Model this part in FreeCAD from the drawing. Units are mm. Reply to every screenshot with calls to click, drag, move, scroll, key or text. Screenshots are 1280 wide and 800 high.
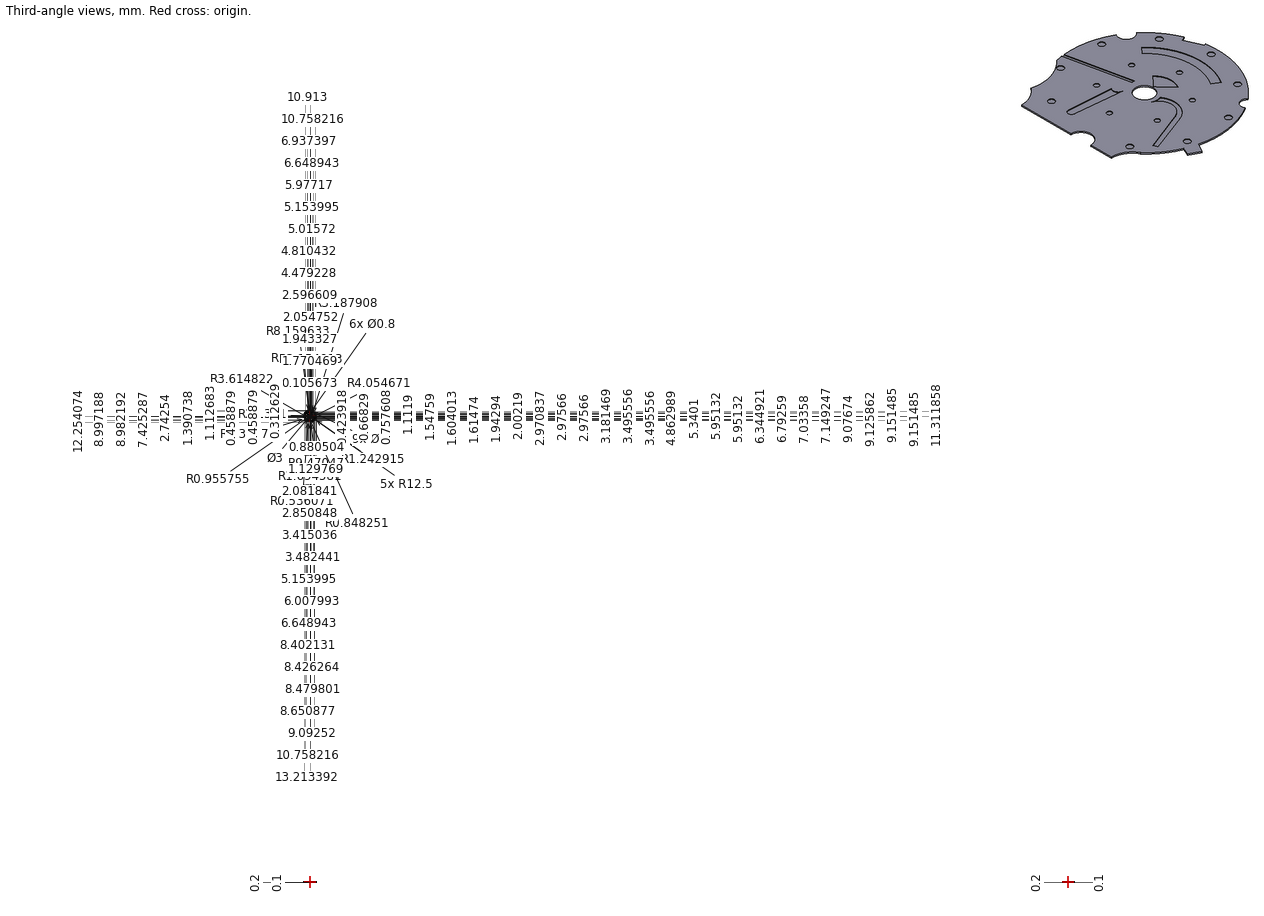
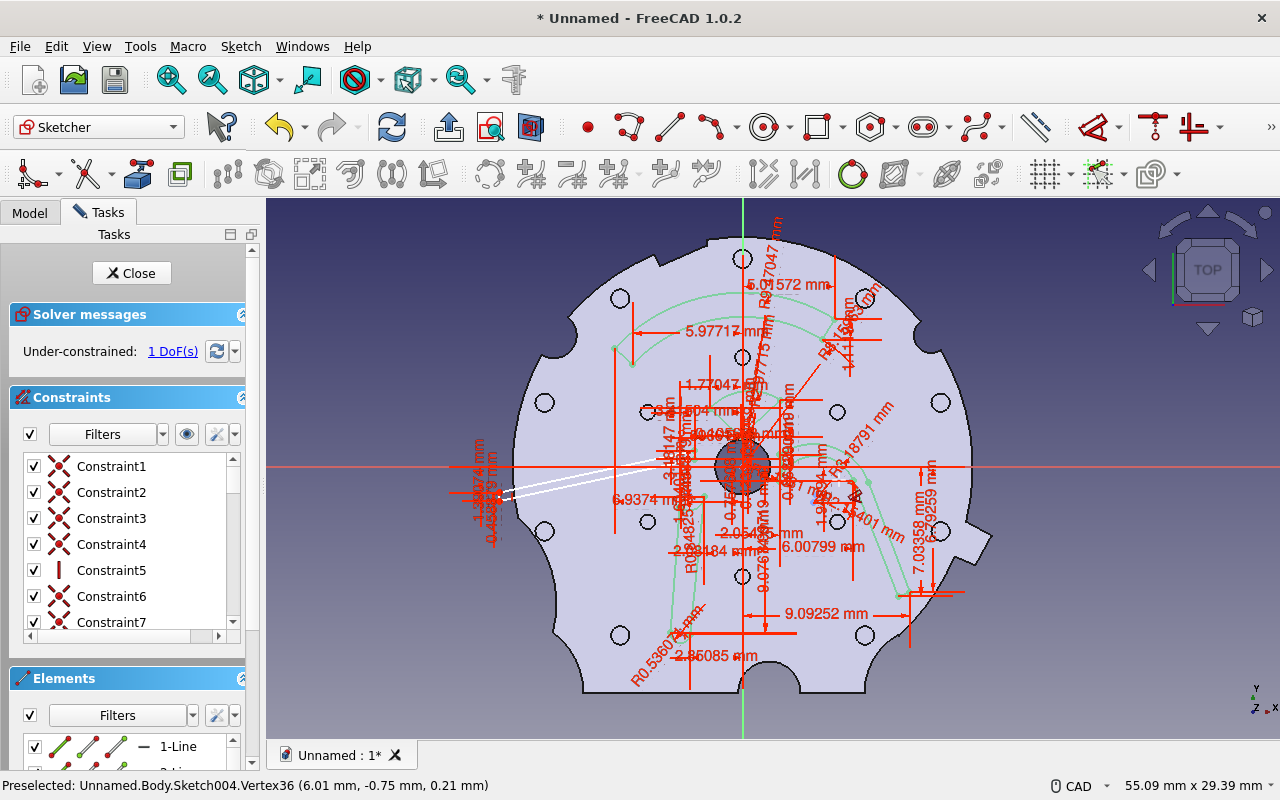
scroll(499, 493, up, 2)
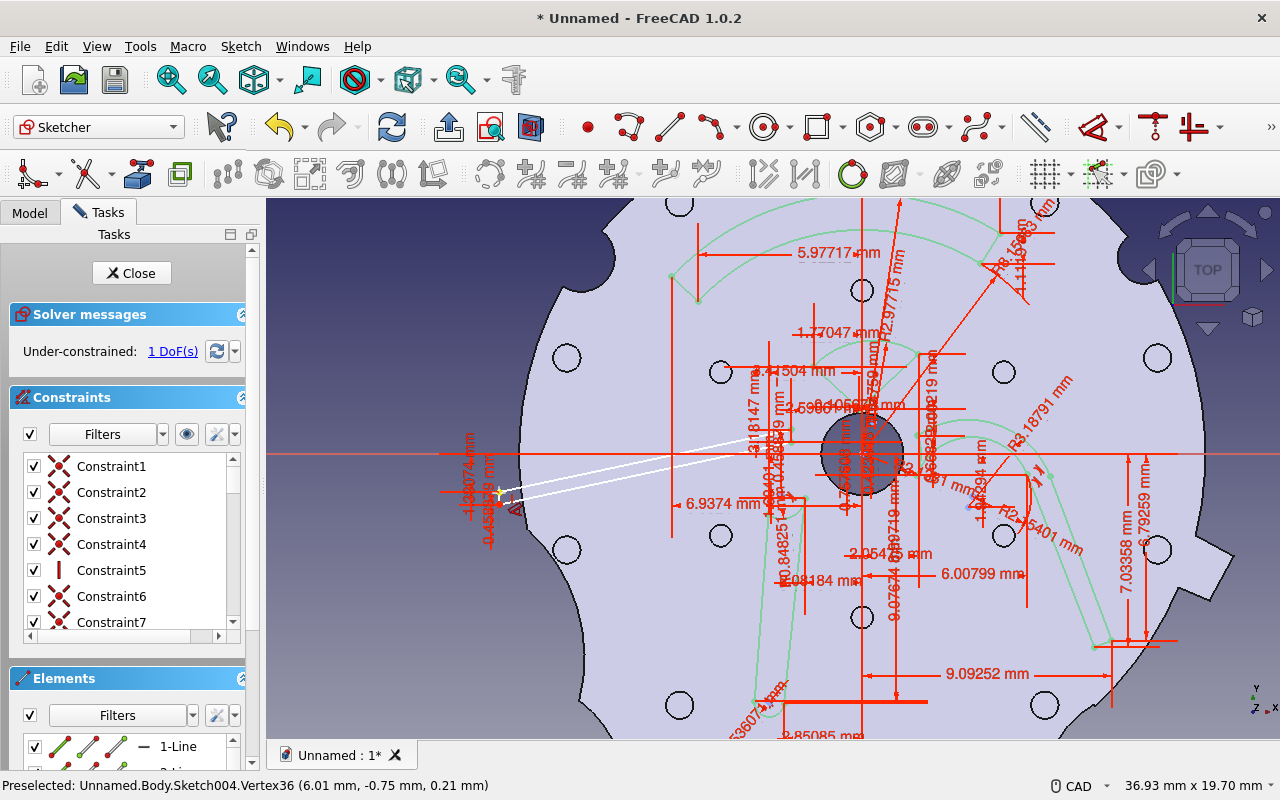
click(499, 492)
click(681, 526)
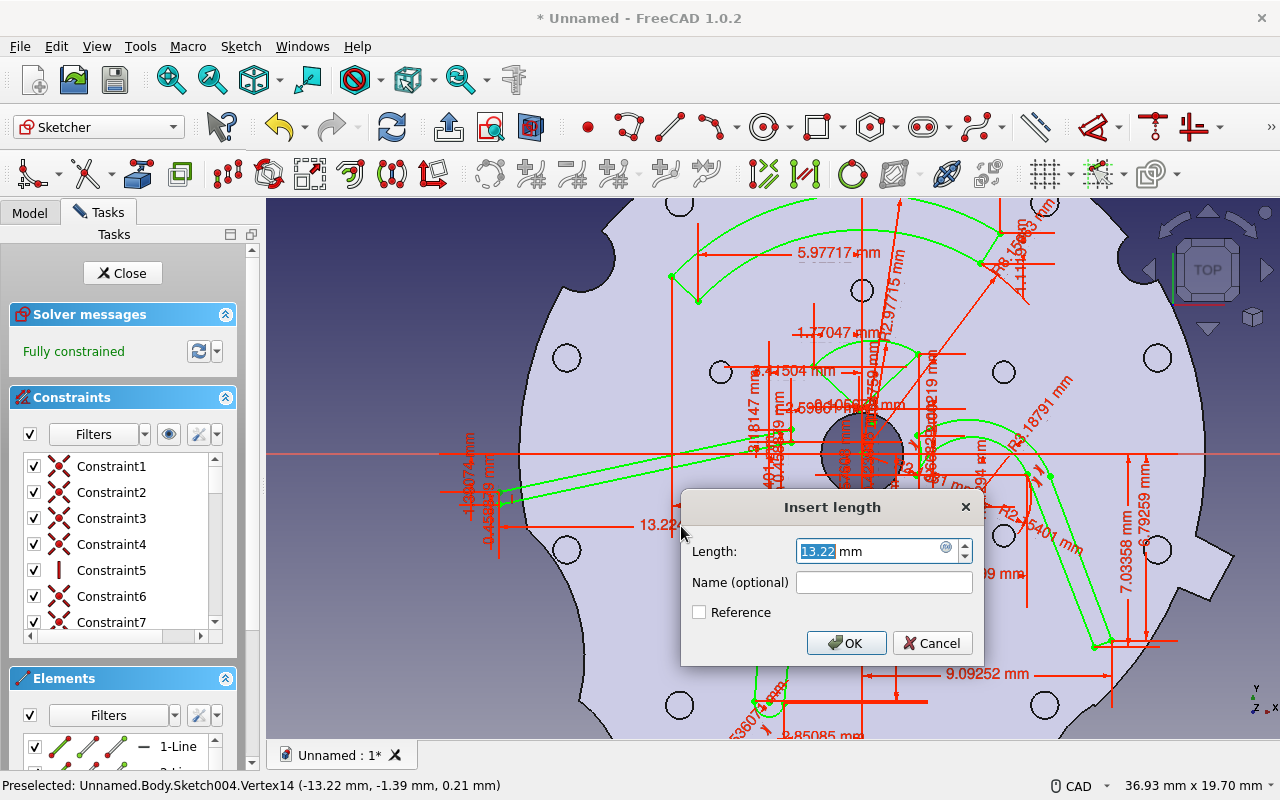
text(13.213392)
key(Return)
key(Escape)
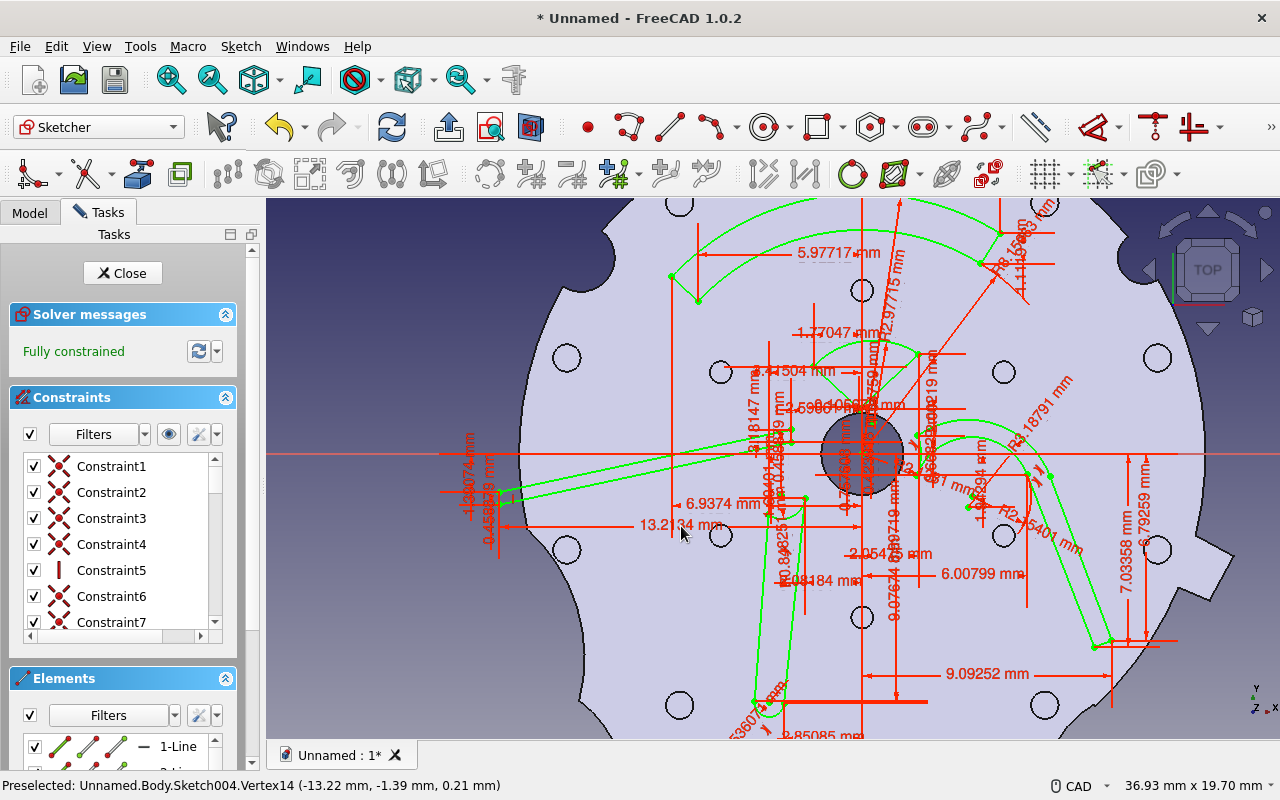
click(123, 273)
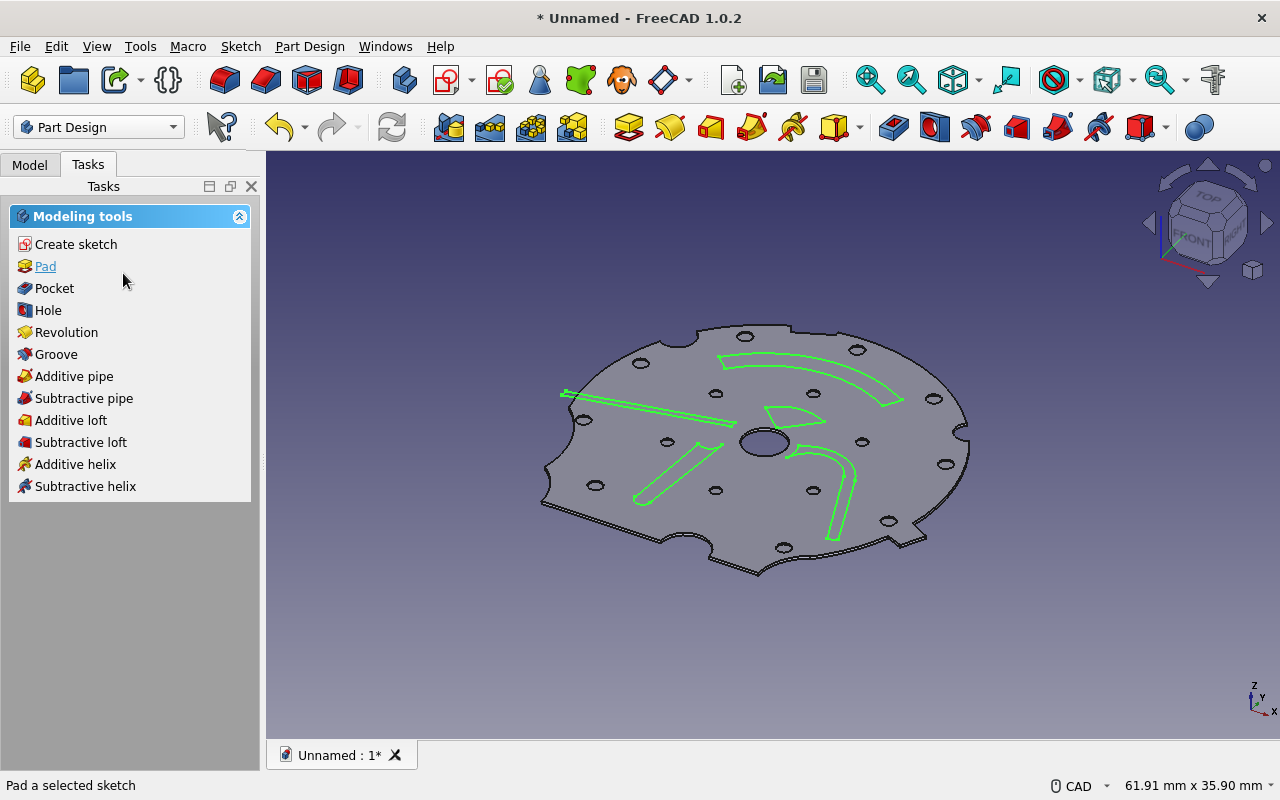
click(894, 128)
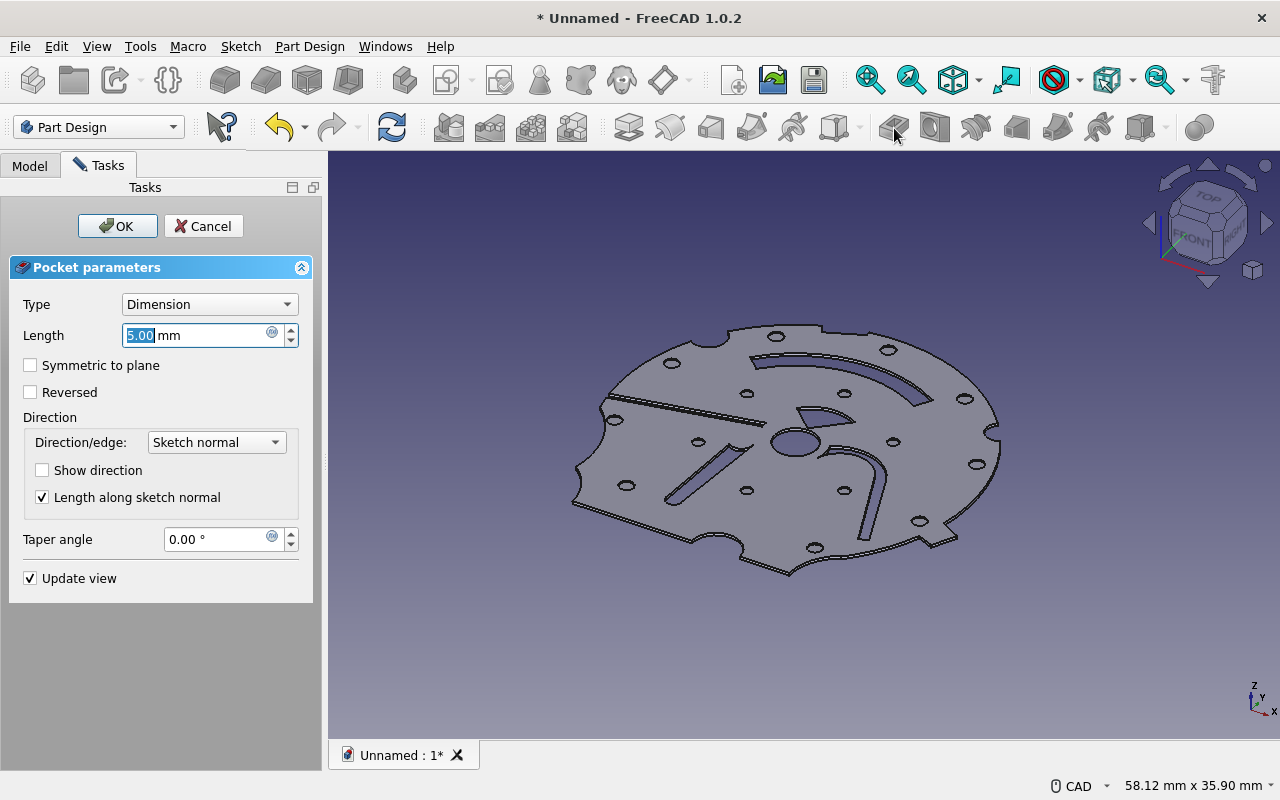
text(0.1)
key(Tab)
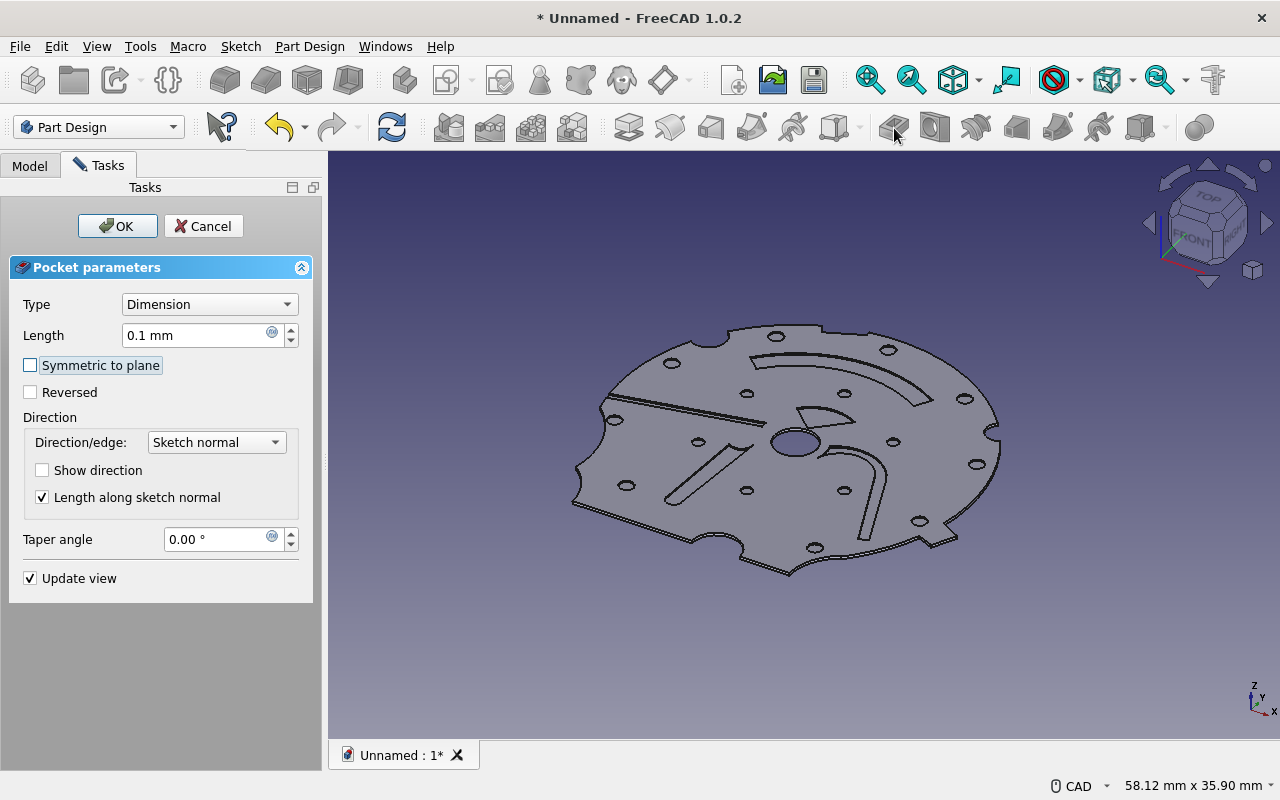
click(118, 226)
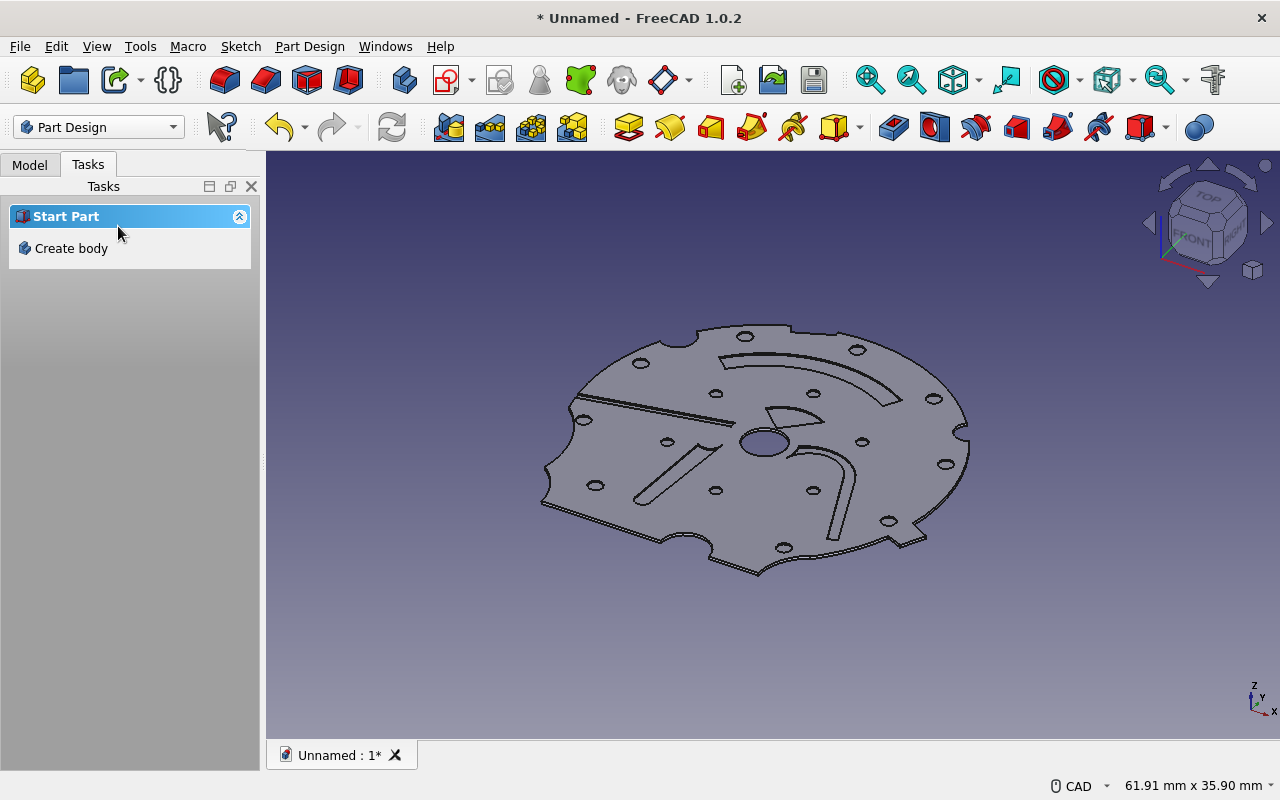
key(0)